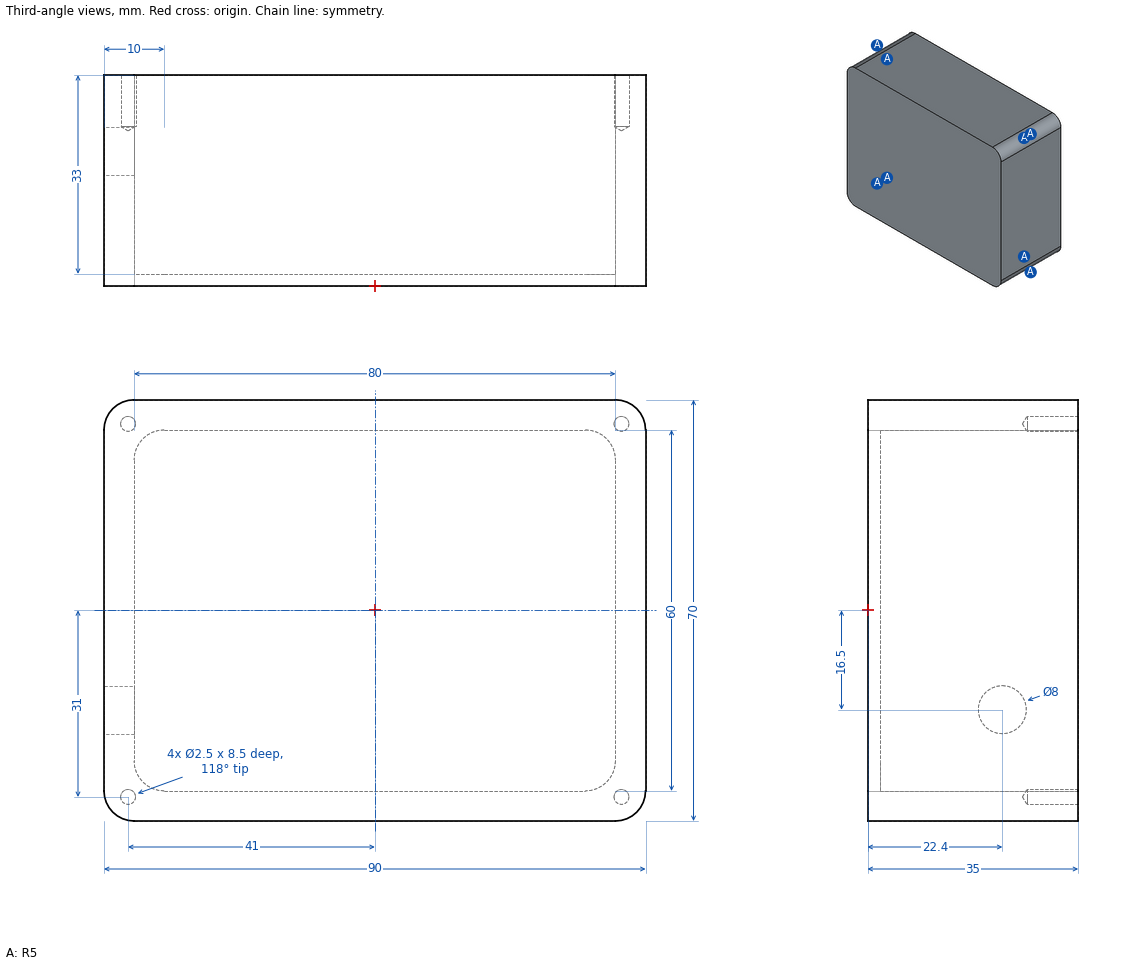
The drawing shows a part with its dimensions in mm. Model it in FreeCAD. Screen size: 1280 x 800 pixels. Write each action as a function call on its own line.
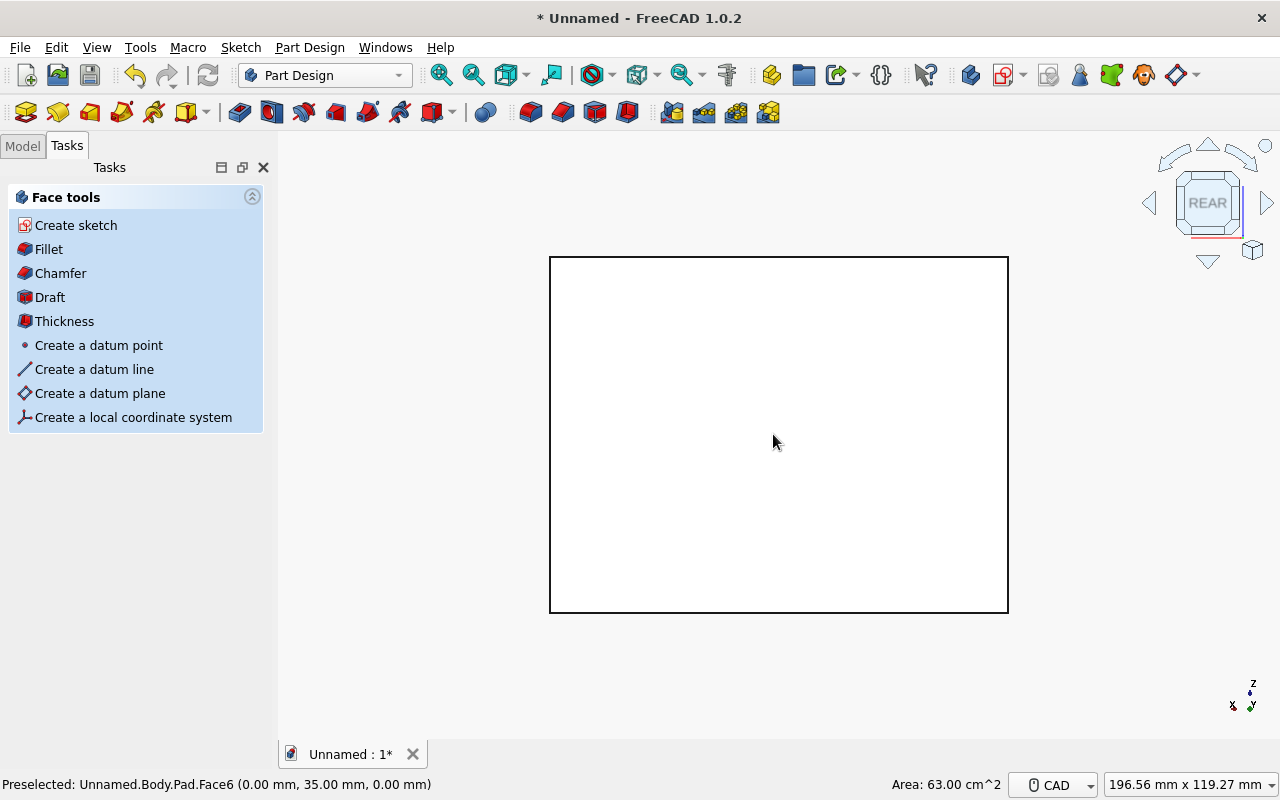
click(1004, 76)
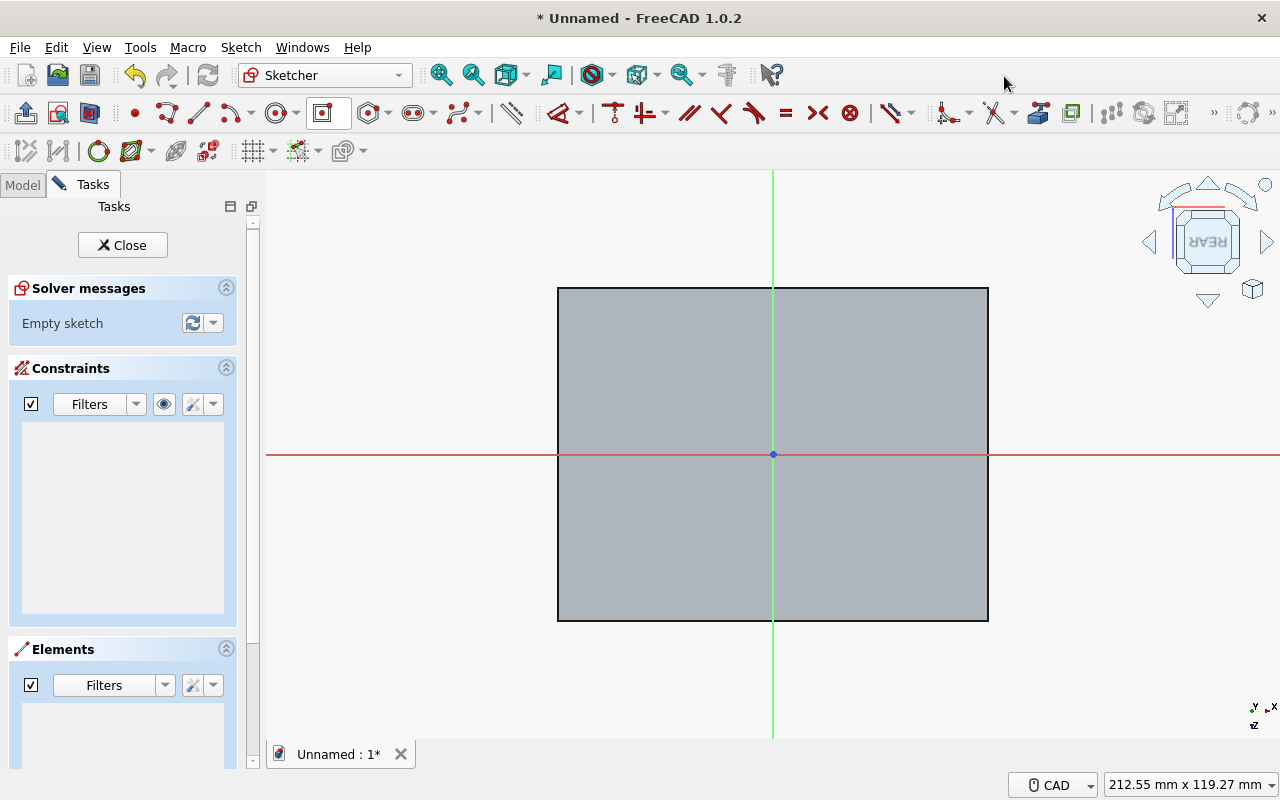
click(322, 114)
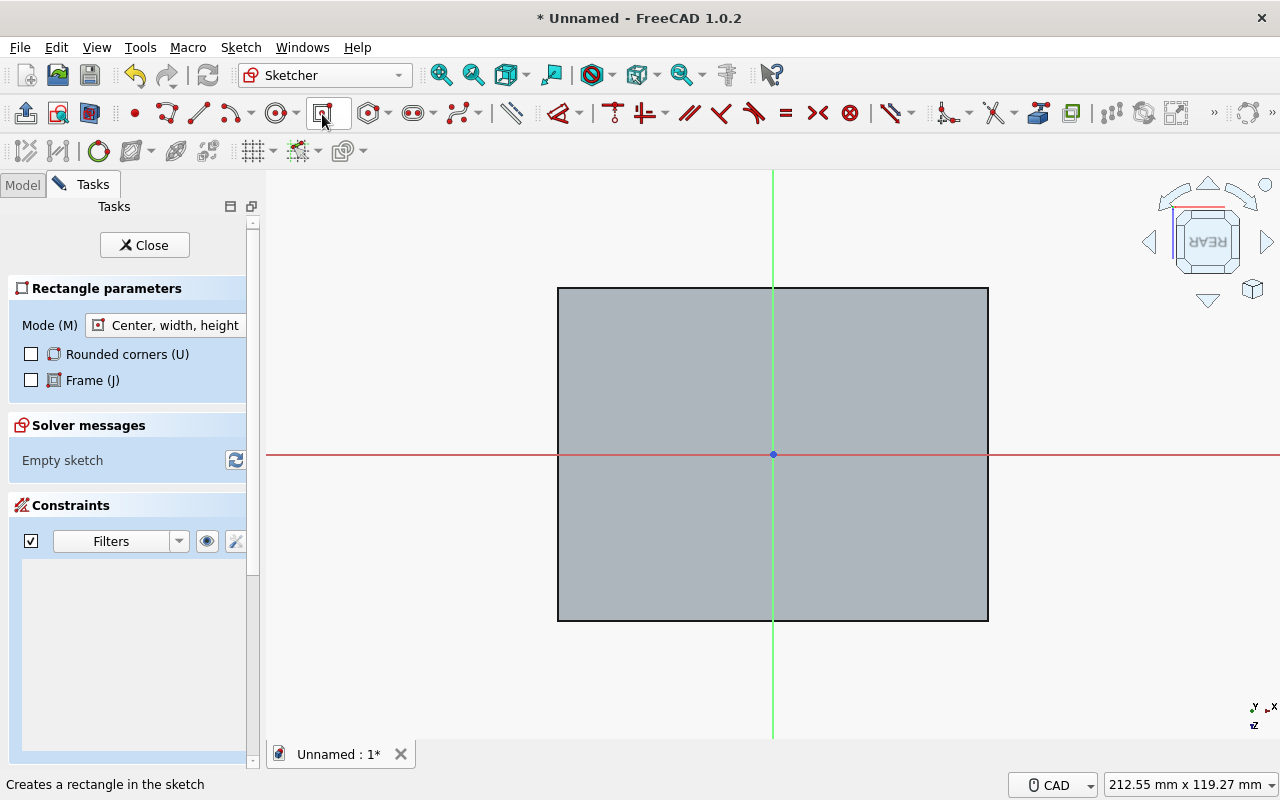
click(773, 455)
click(964, 311)
key(Escape)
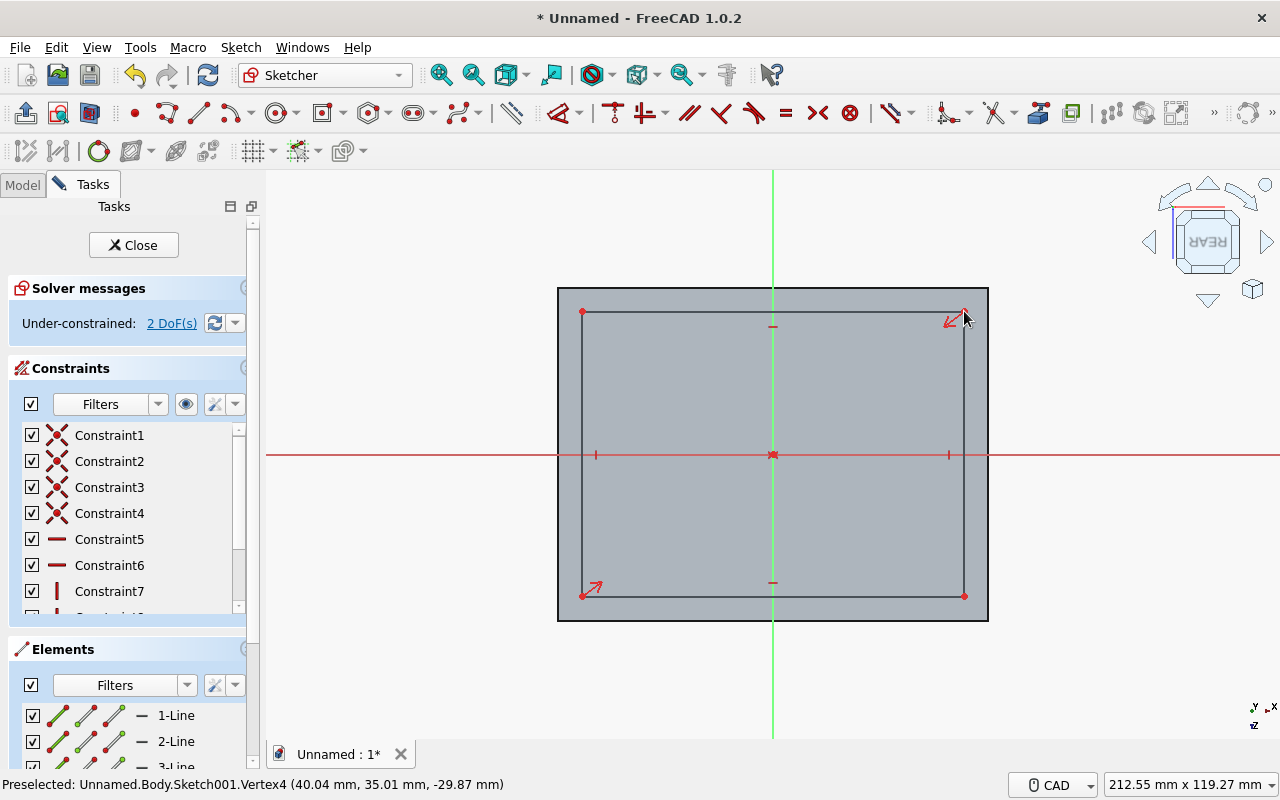
click(558, 114)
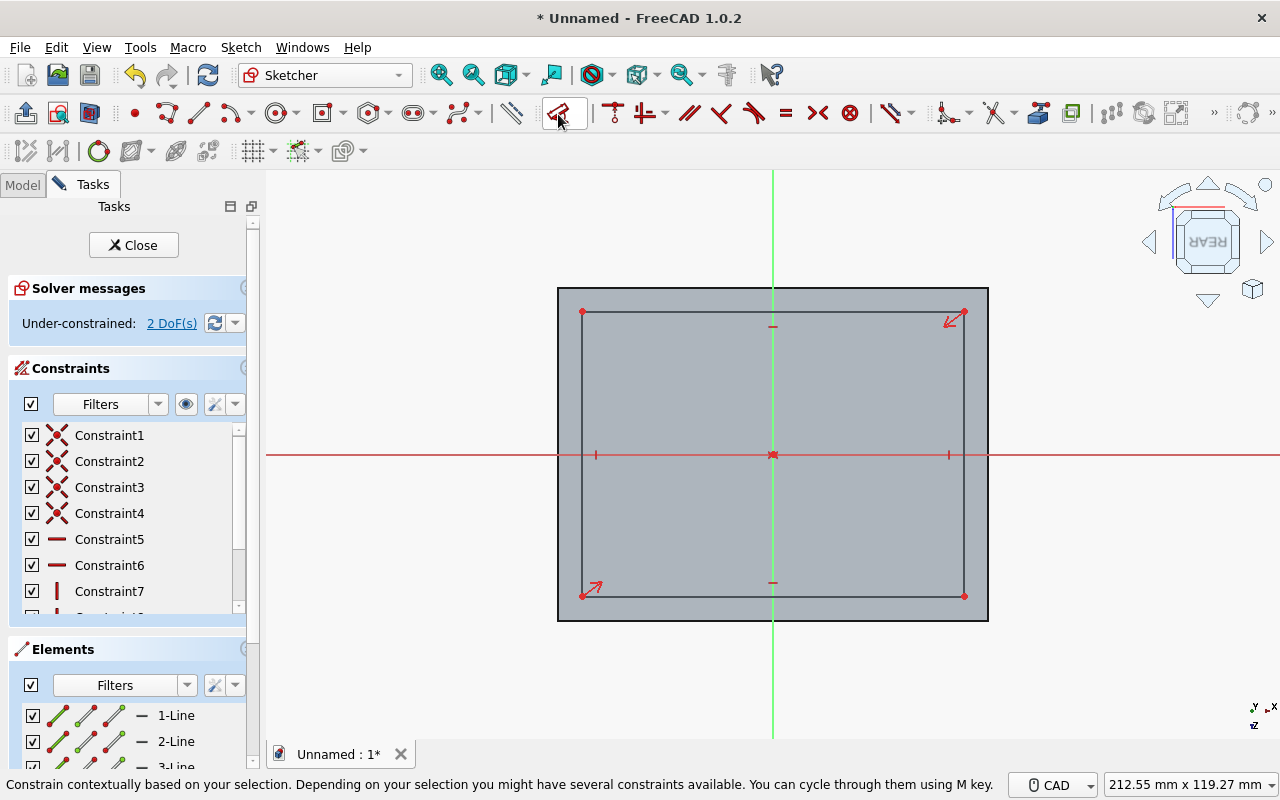
click(697, 597)
click(685, 631)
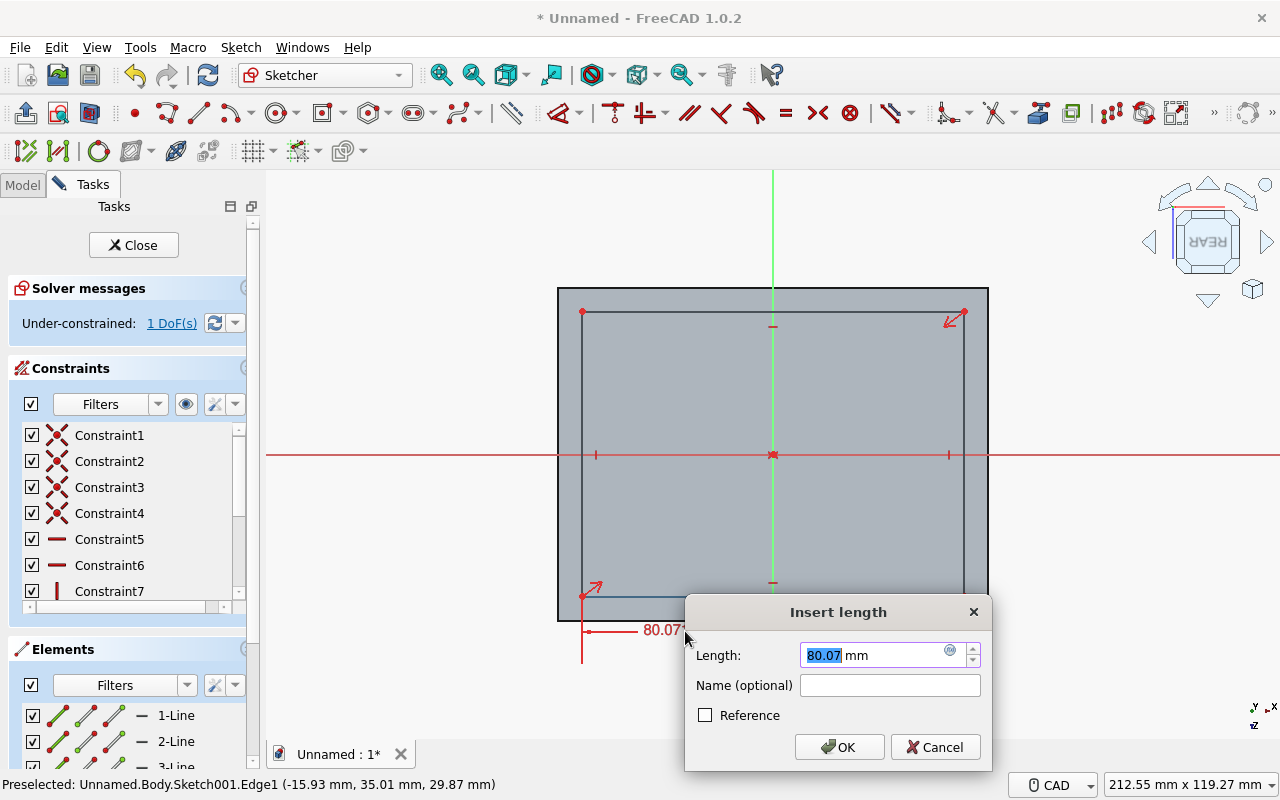
text(80)
key(Return)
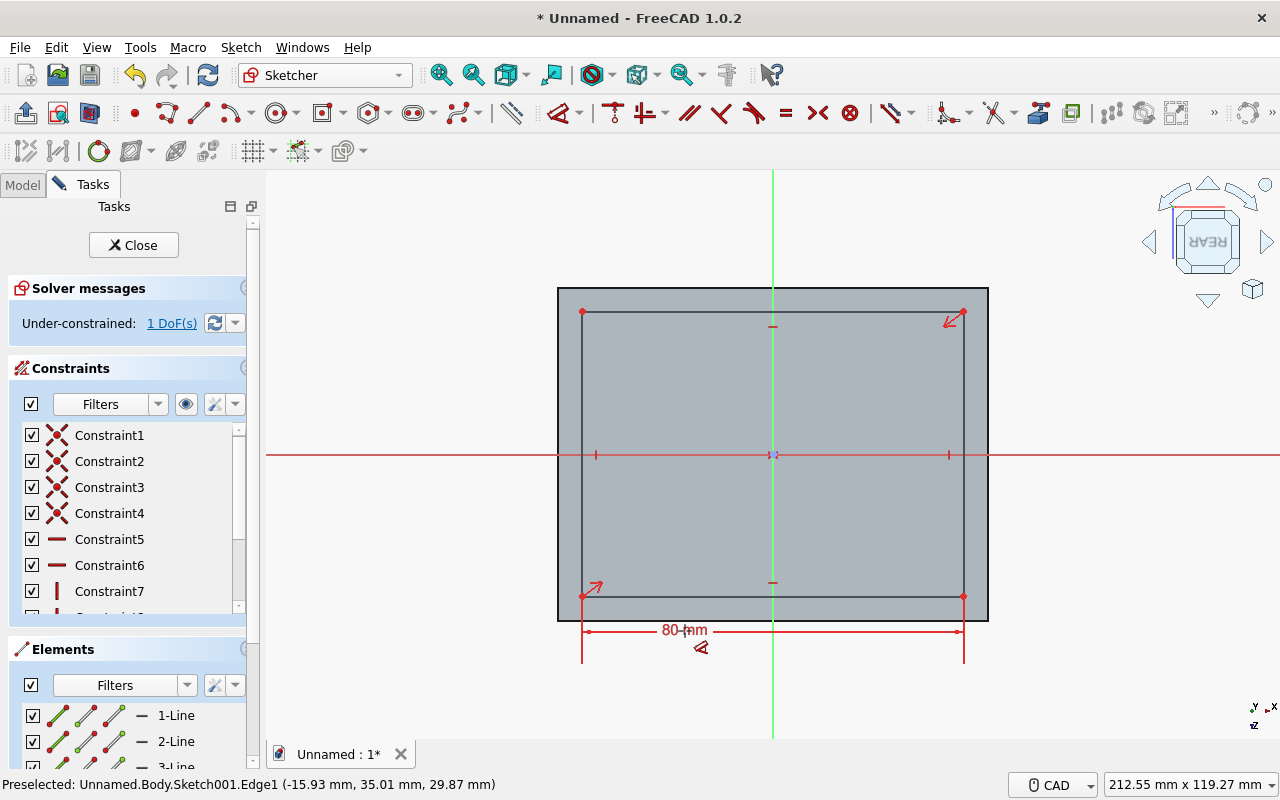
click(964, 512)
click(998, 389)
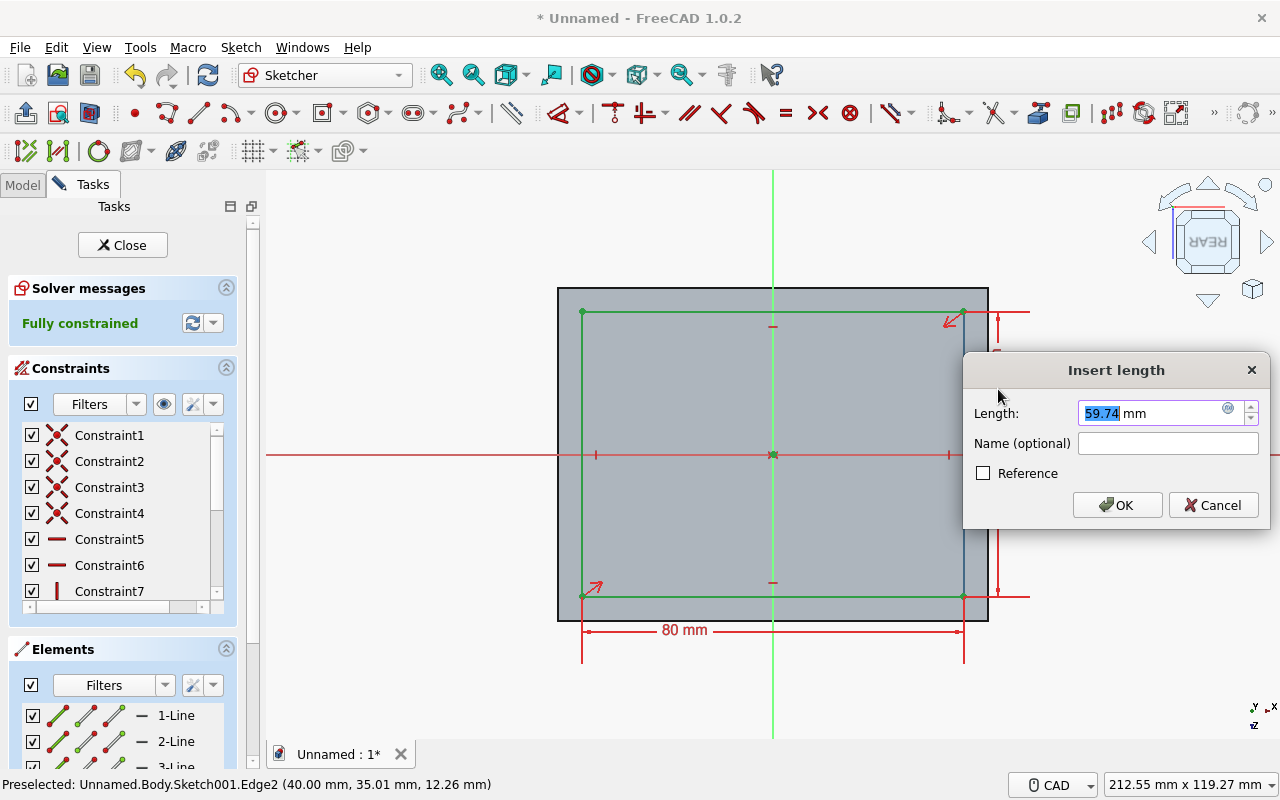
text(60)
key(Return)
key(Escape)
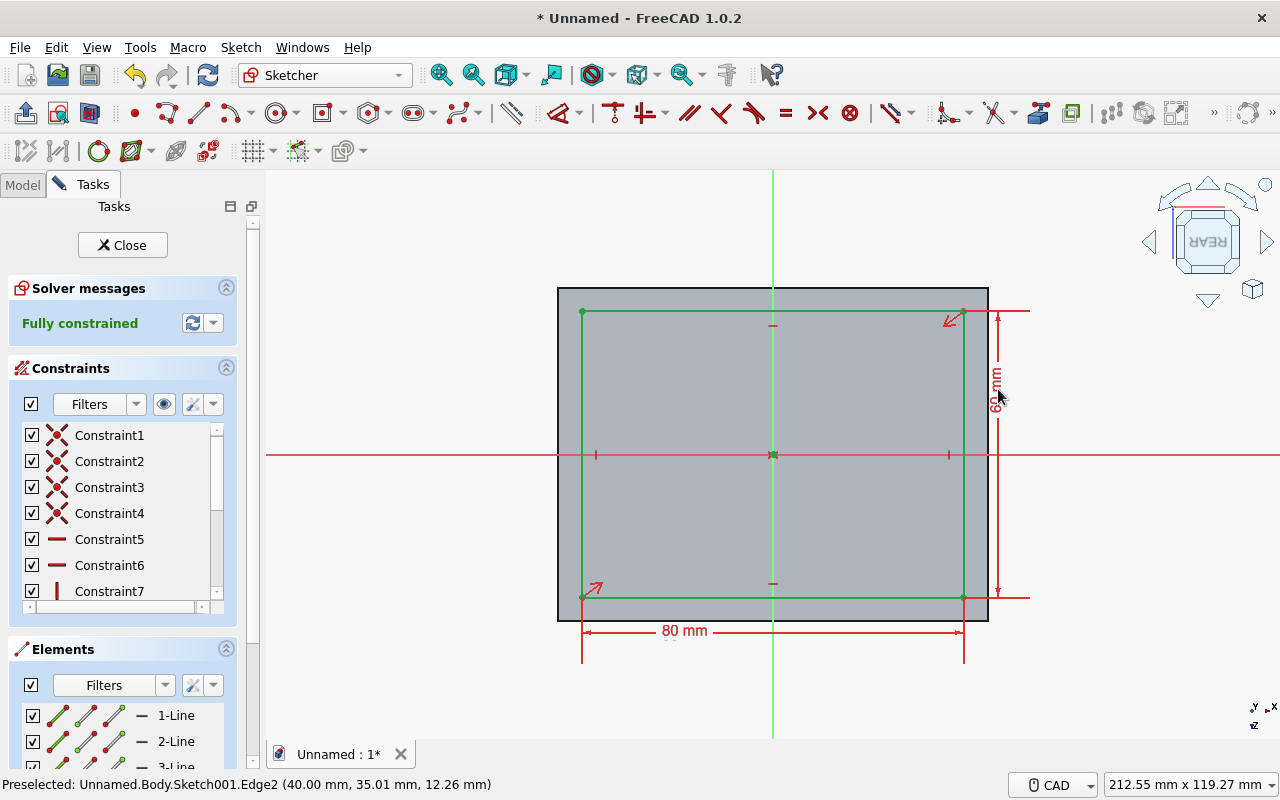
click(123, 245)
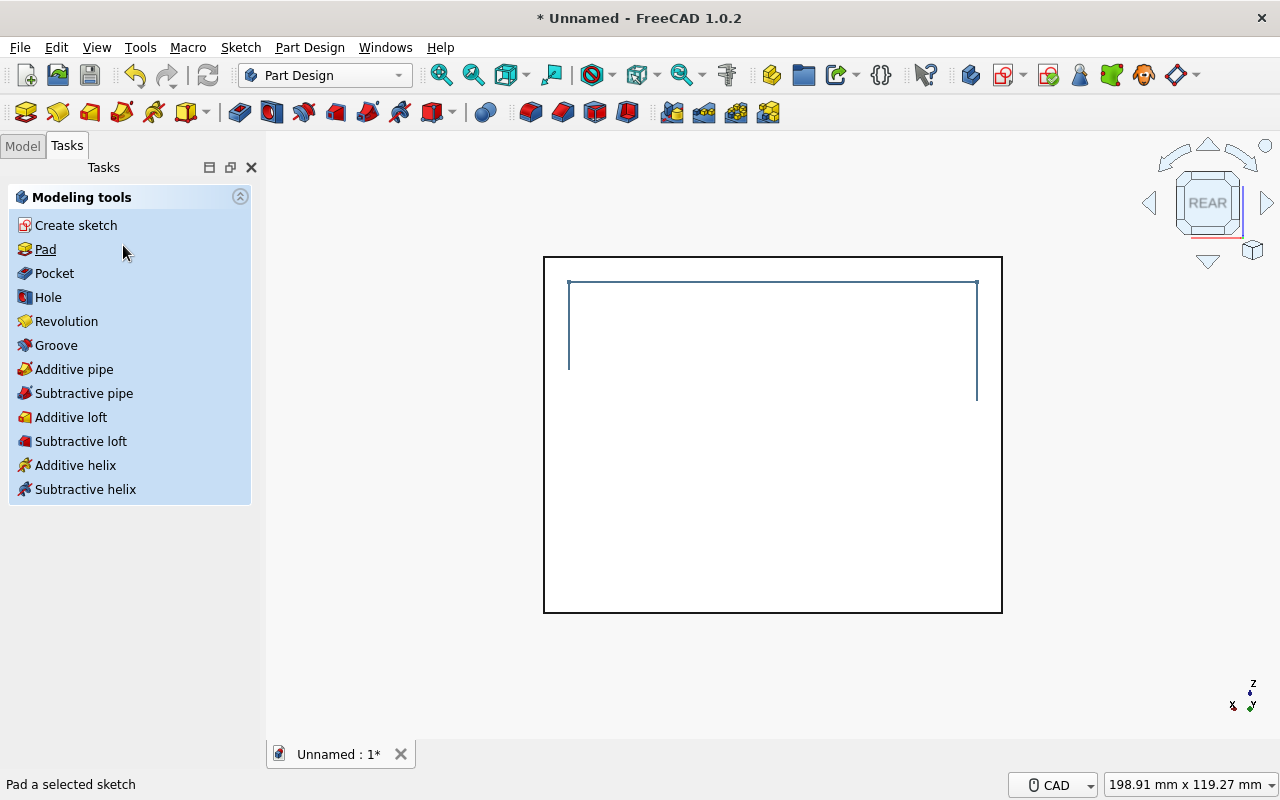
click(240, 112)